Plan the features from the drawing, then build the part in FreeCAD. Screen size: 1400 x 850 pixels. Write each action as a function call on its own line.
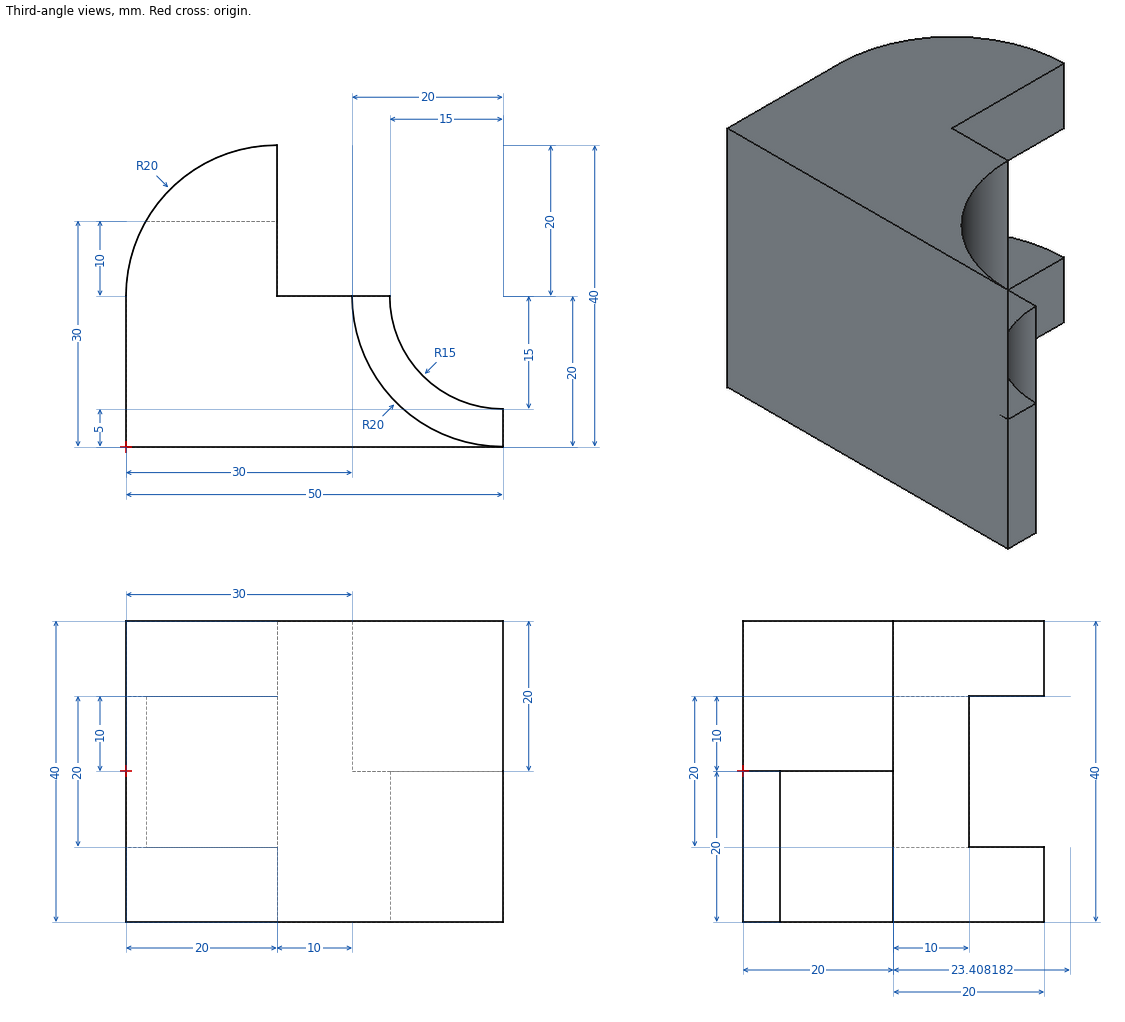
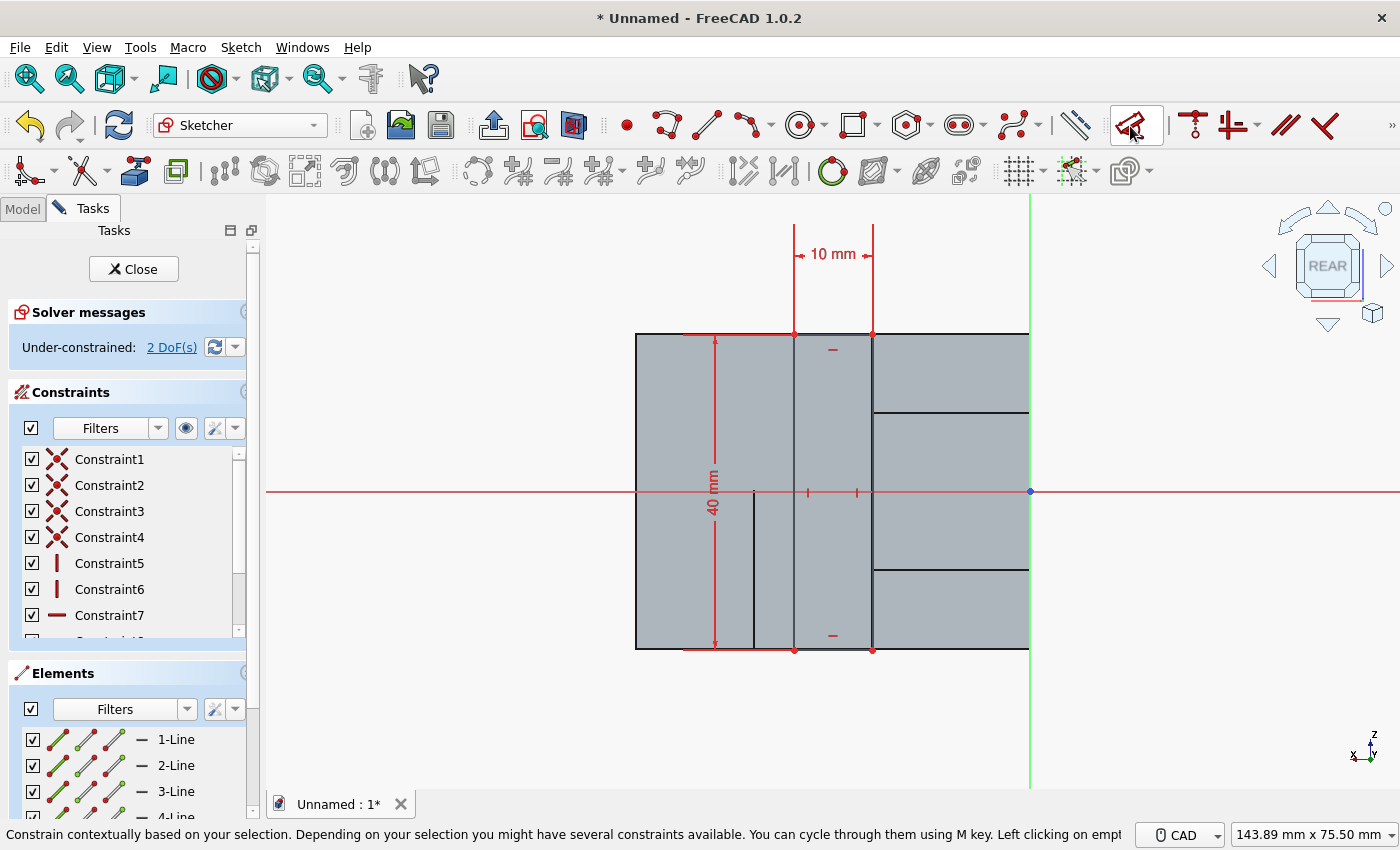
click(794, 335)
click(912, 301)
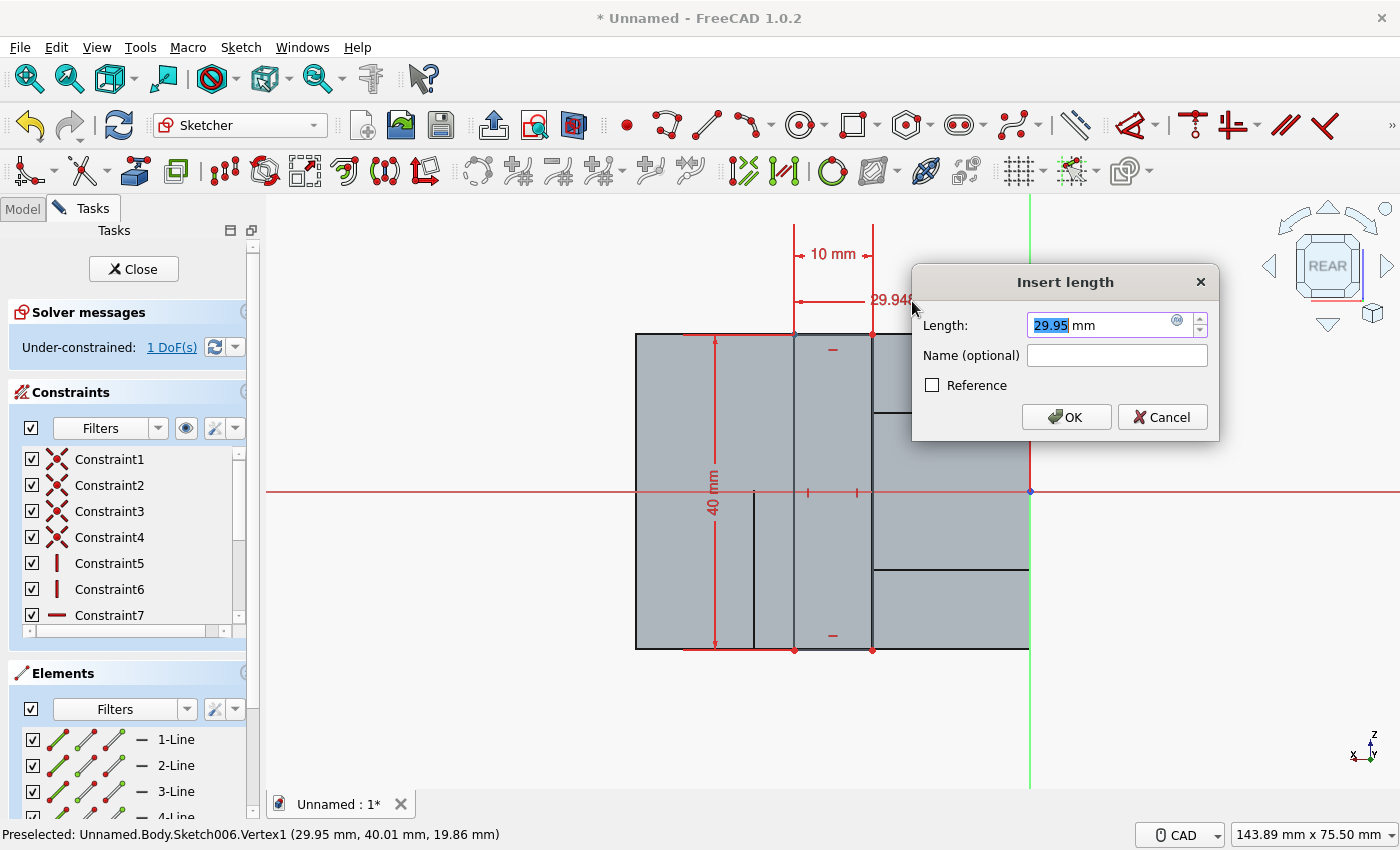
text(30)
key(Return)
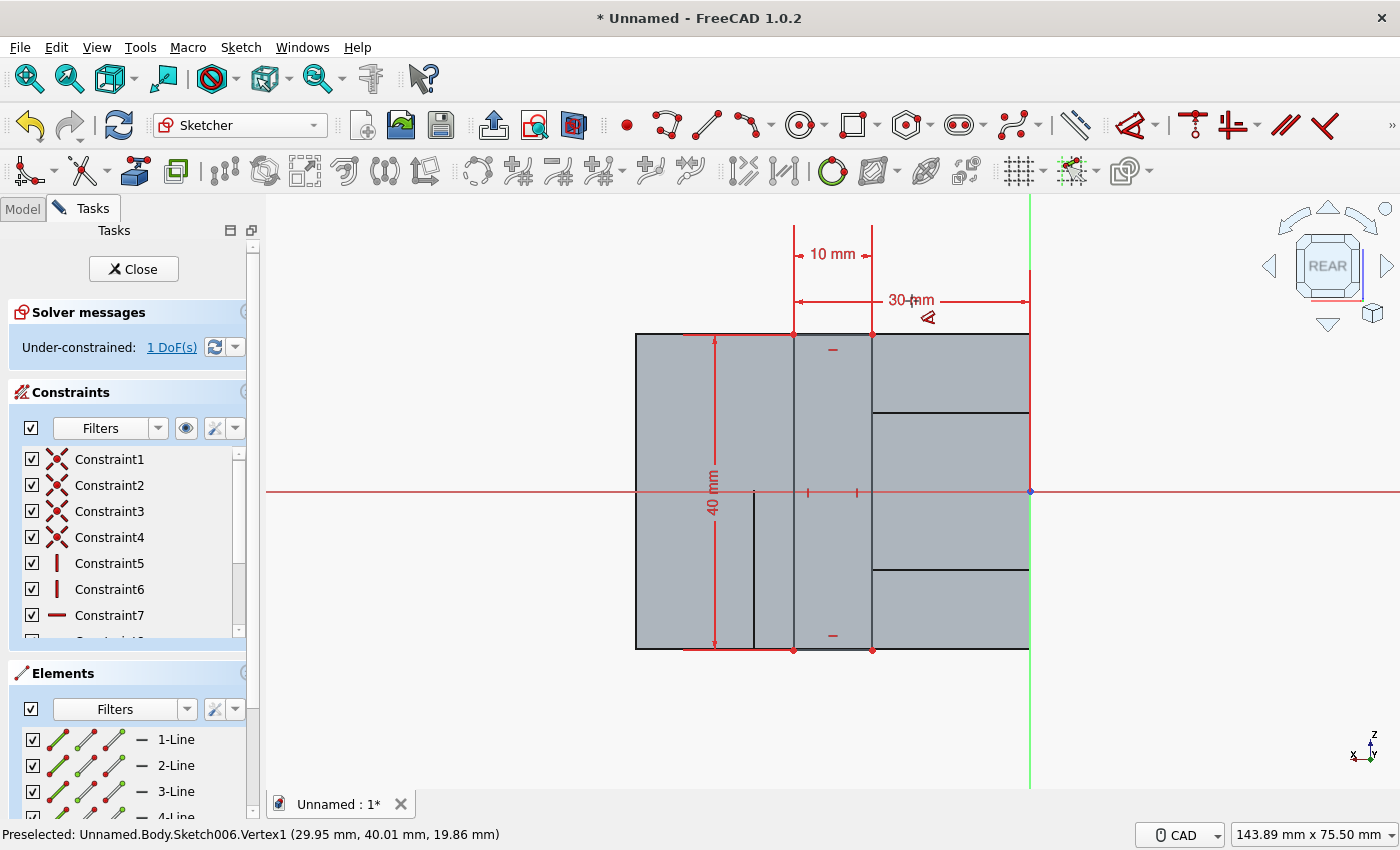
click(794, 335)
click(1064, 413)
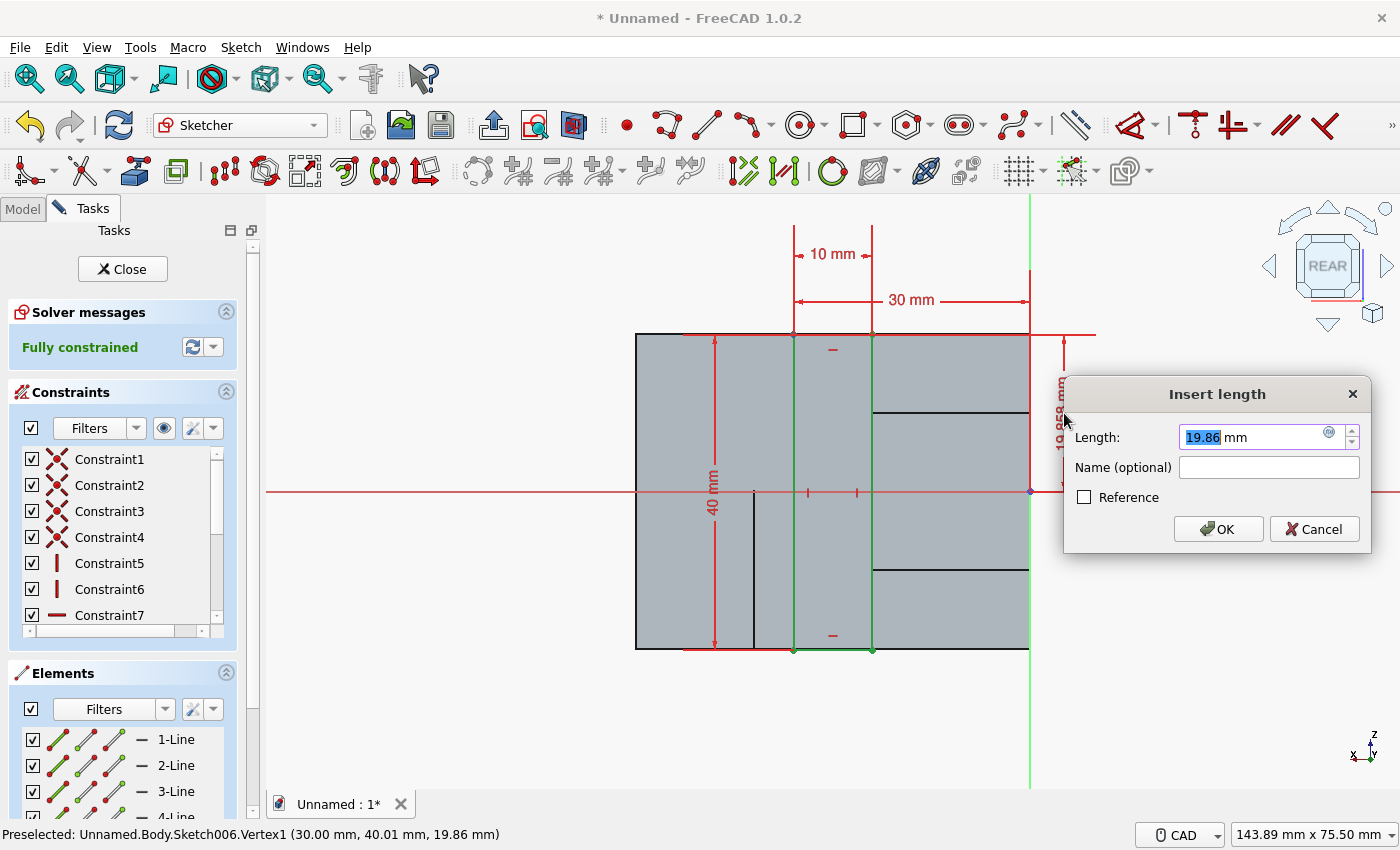
text(20)
key(Return)
key(Escape)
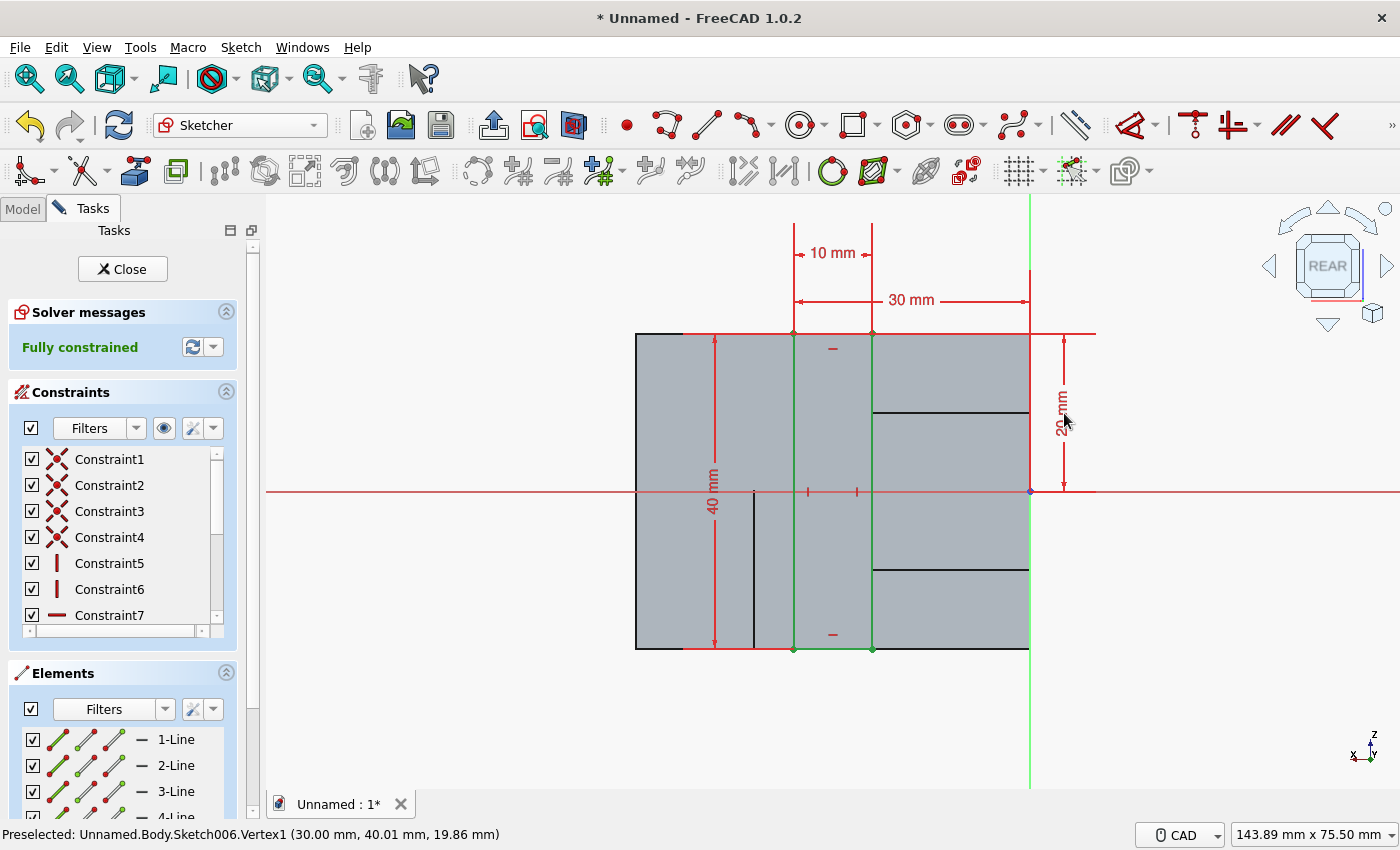
click(123, 269)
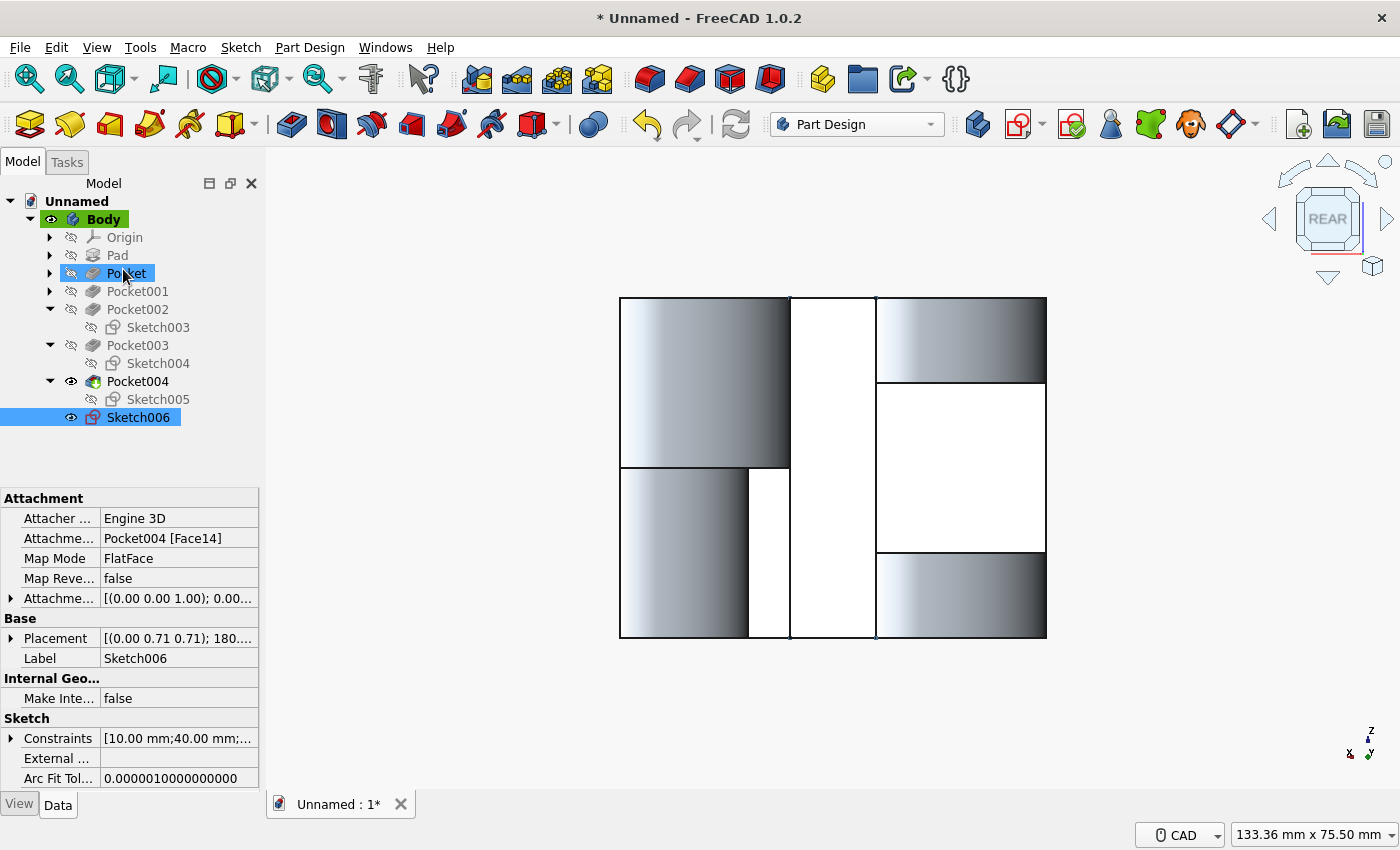
click(292, 124)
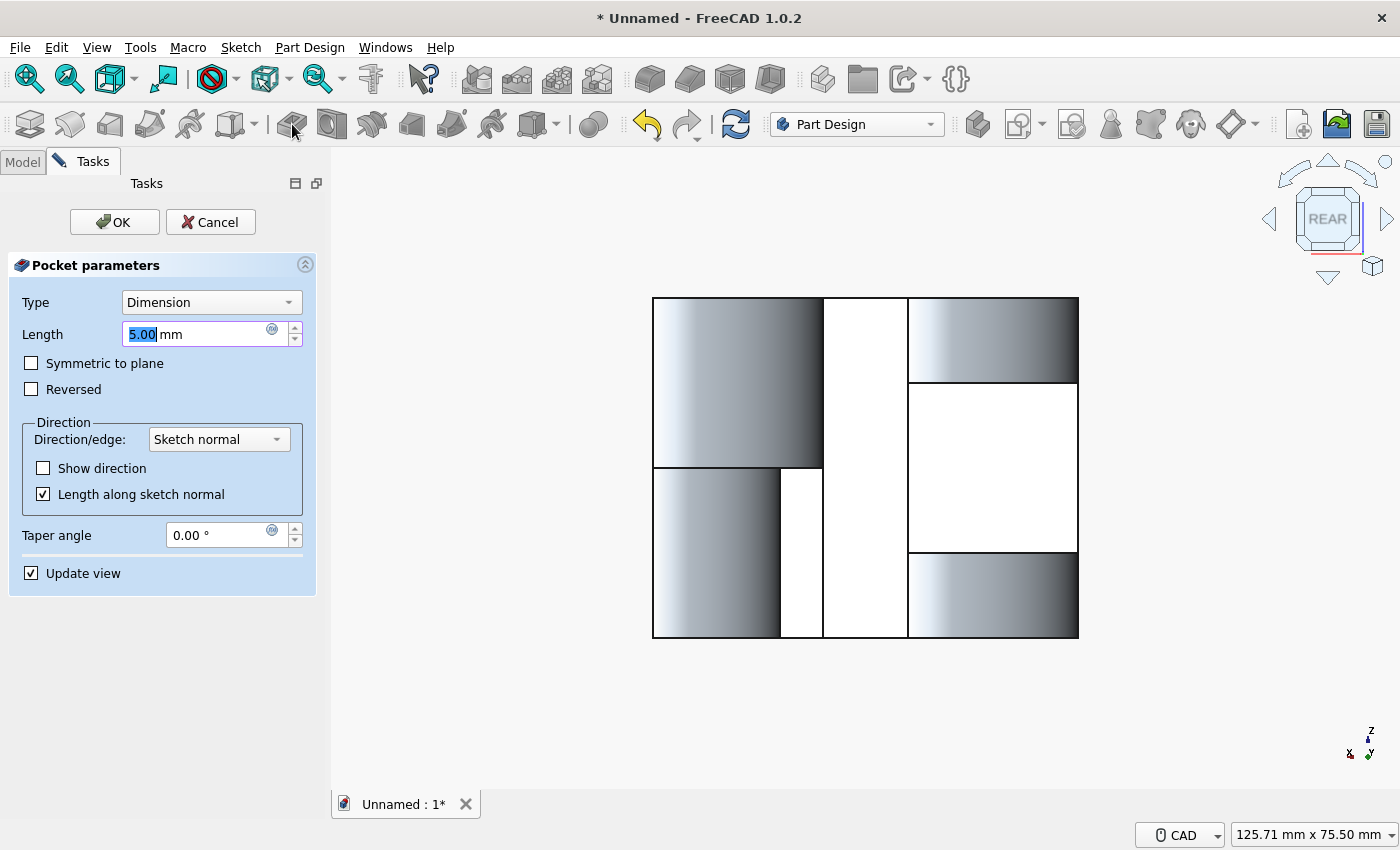
text(20)
key(Tab)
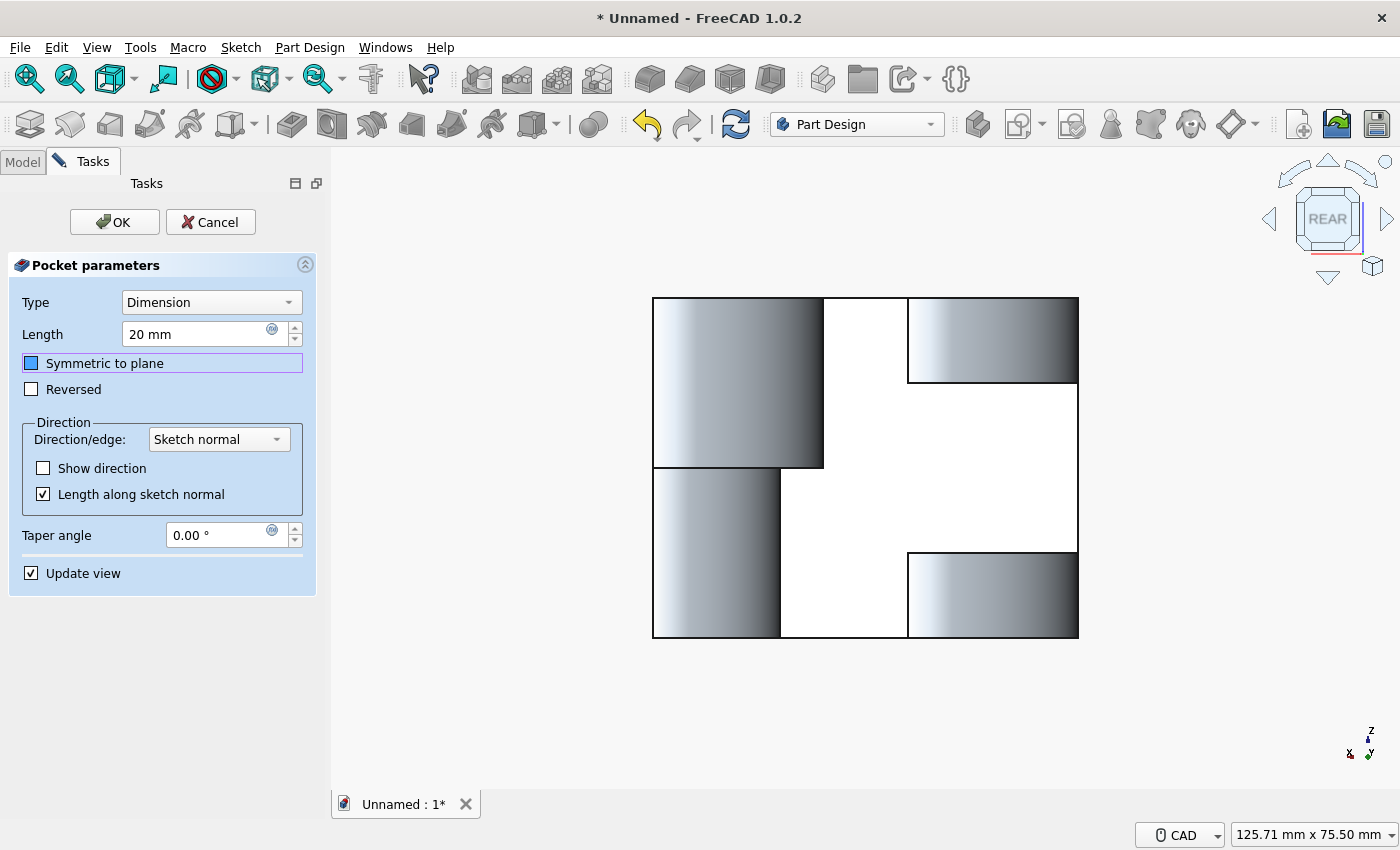
click(115, 222)